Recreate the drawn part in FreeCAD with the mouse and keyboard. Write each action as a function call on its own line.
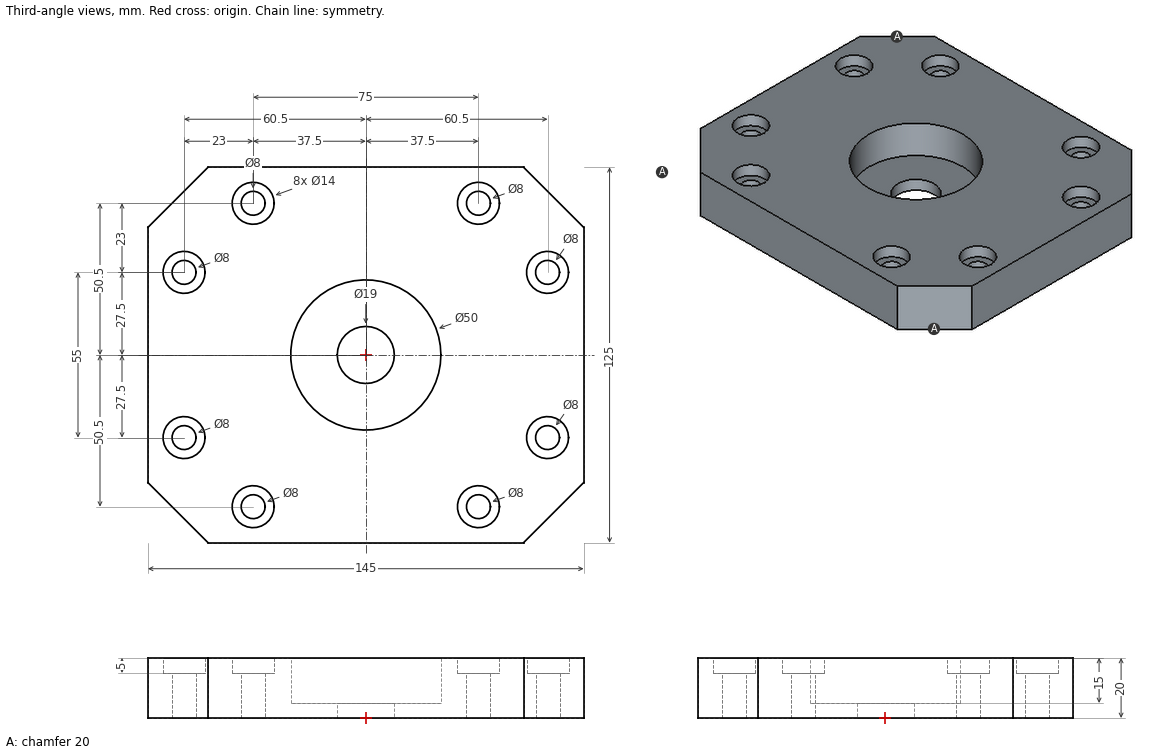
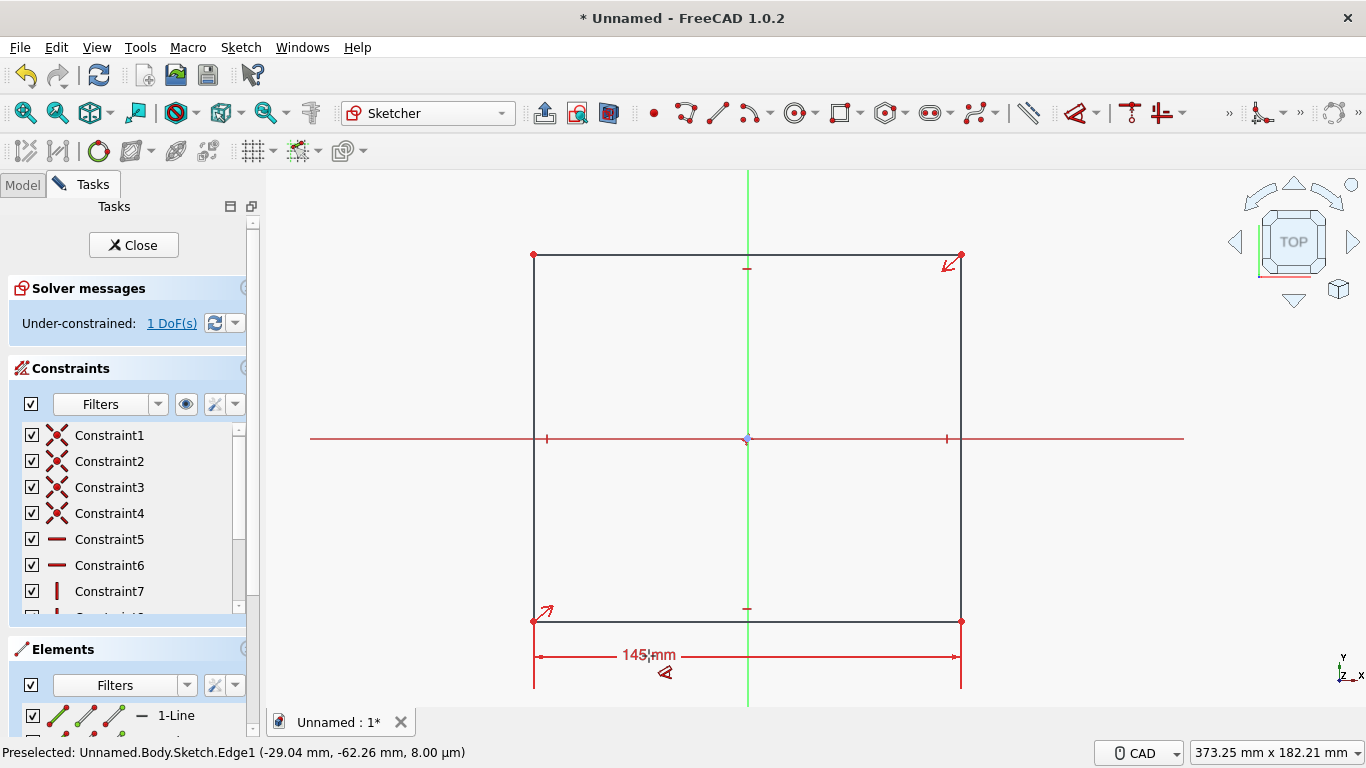
click(961, 512)
click(995, 354)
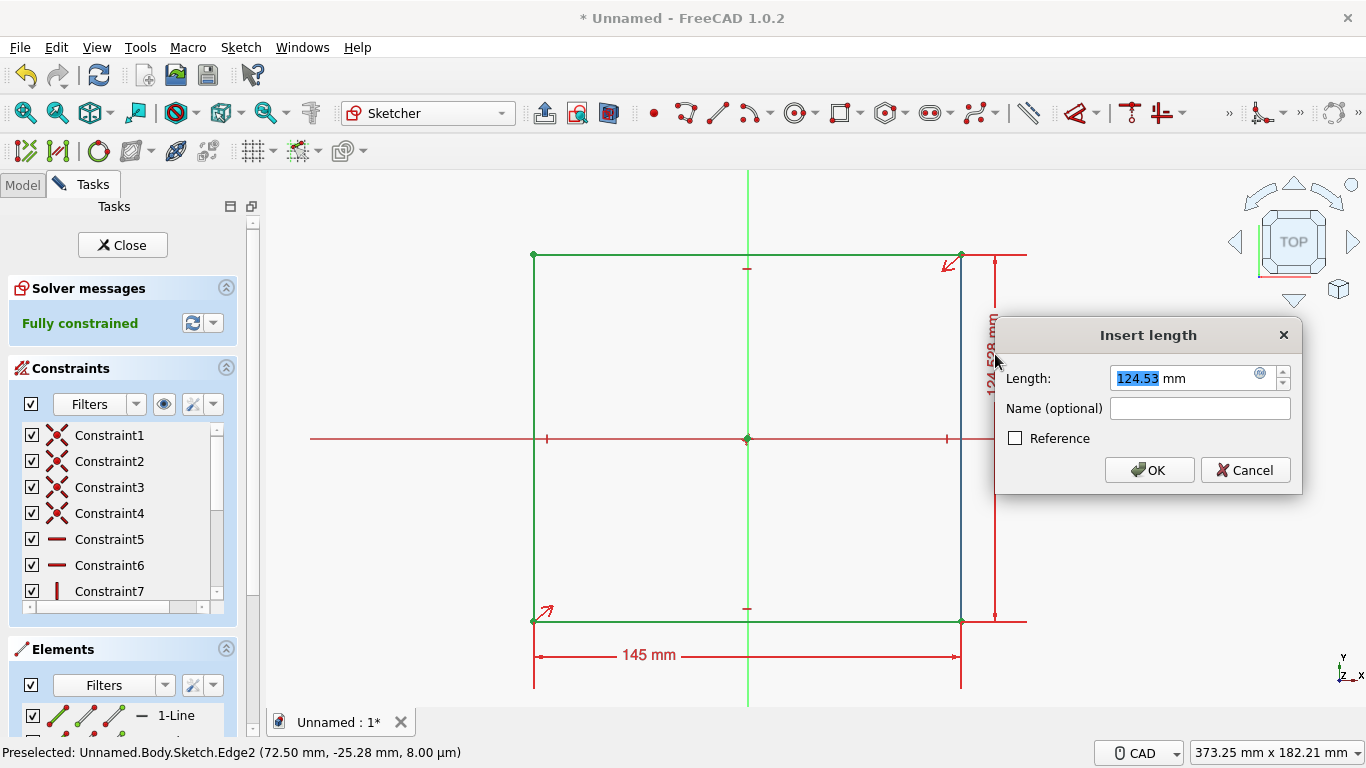
text(125)
key(Return)
key(Escape)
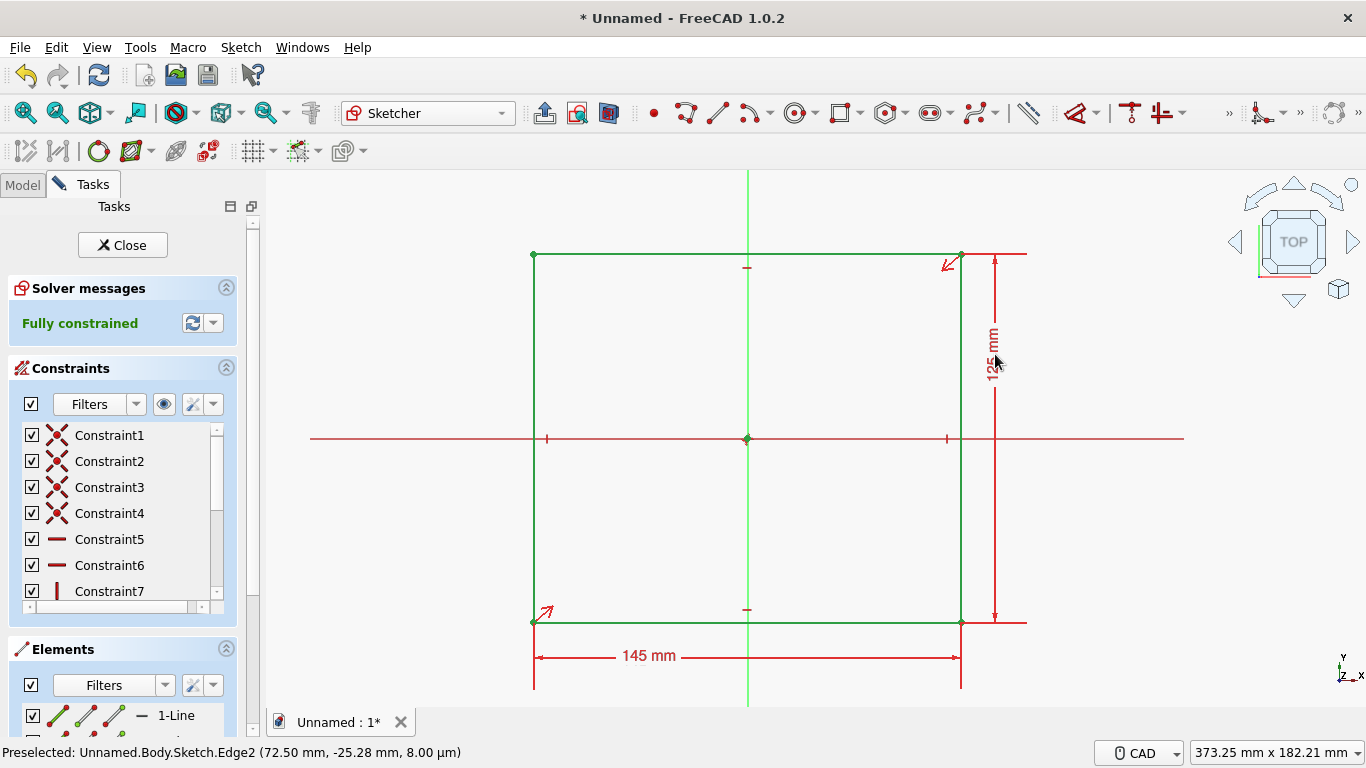
click(123, 245)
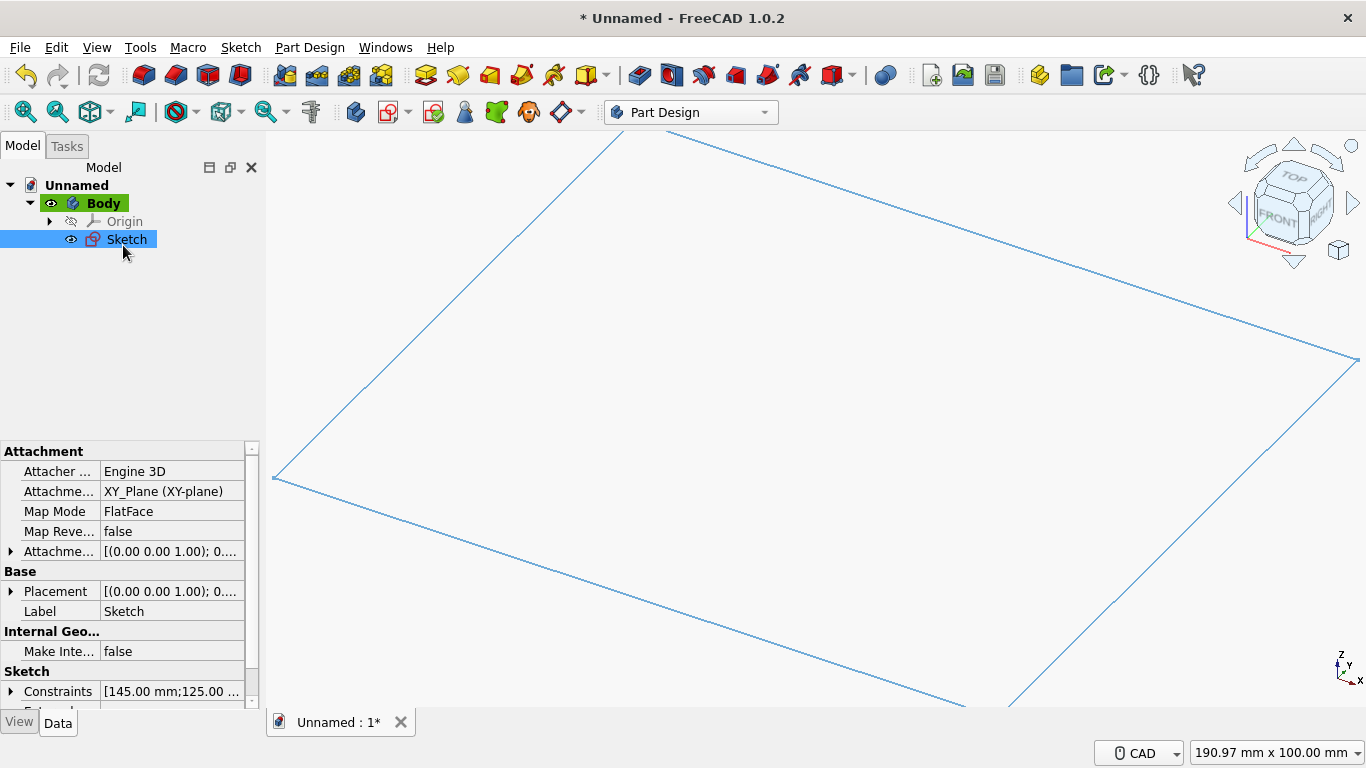
click(426, 76)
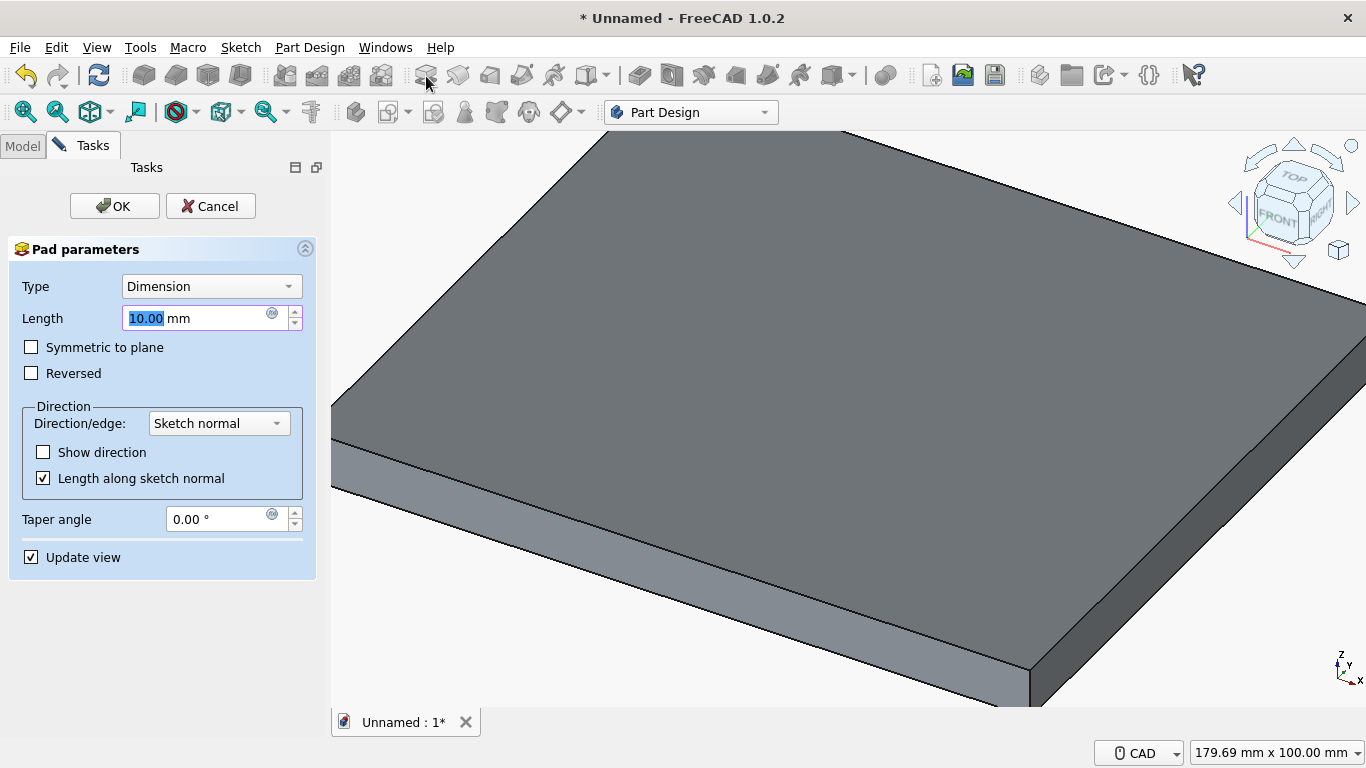
text(20)
key(Tab)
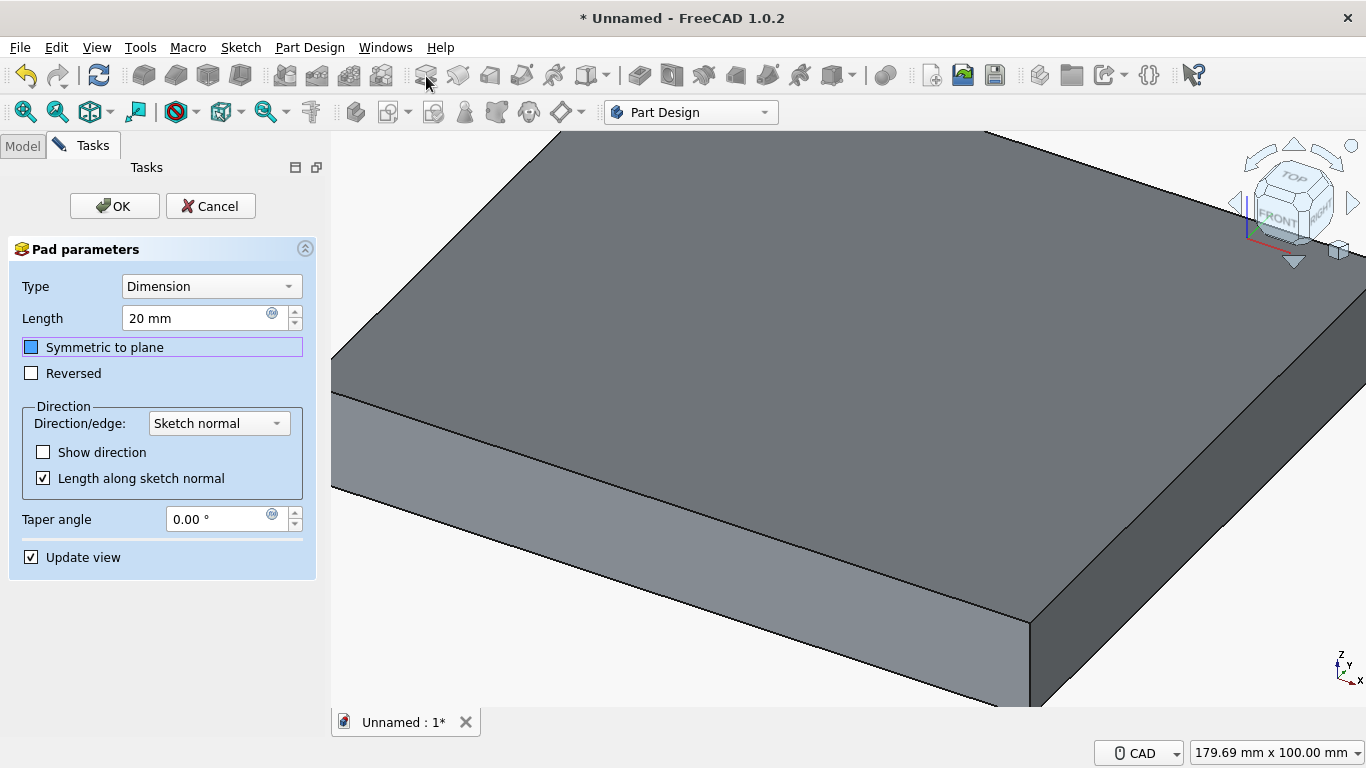
click(115, 206)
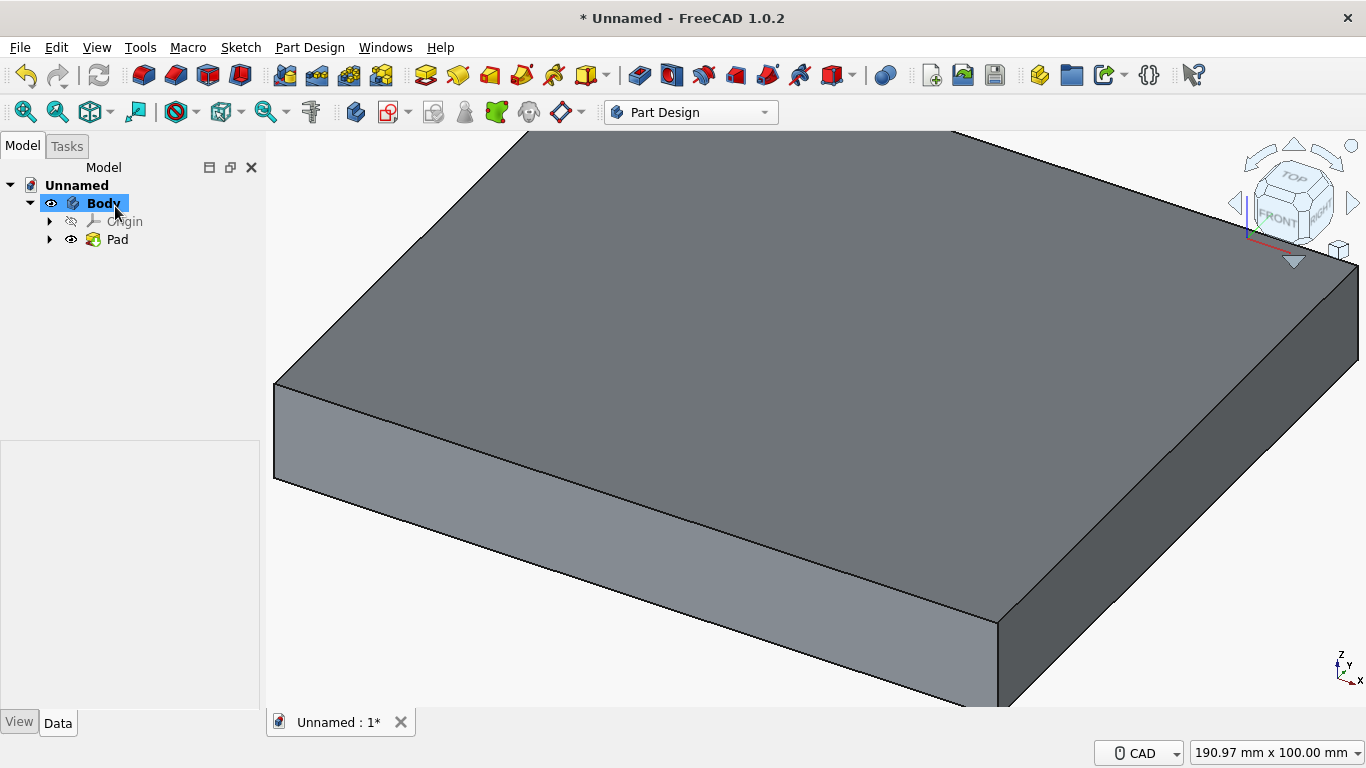
click(26, 112)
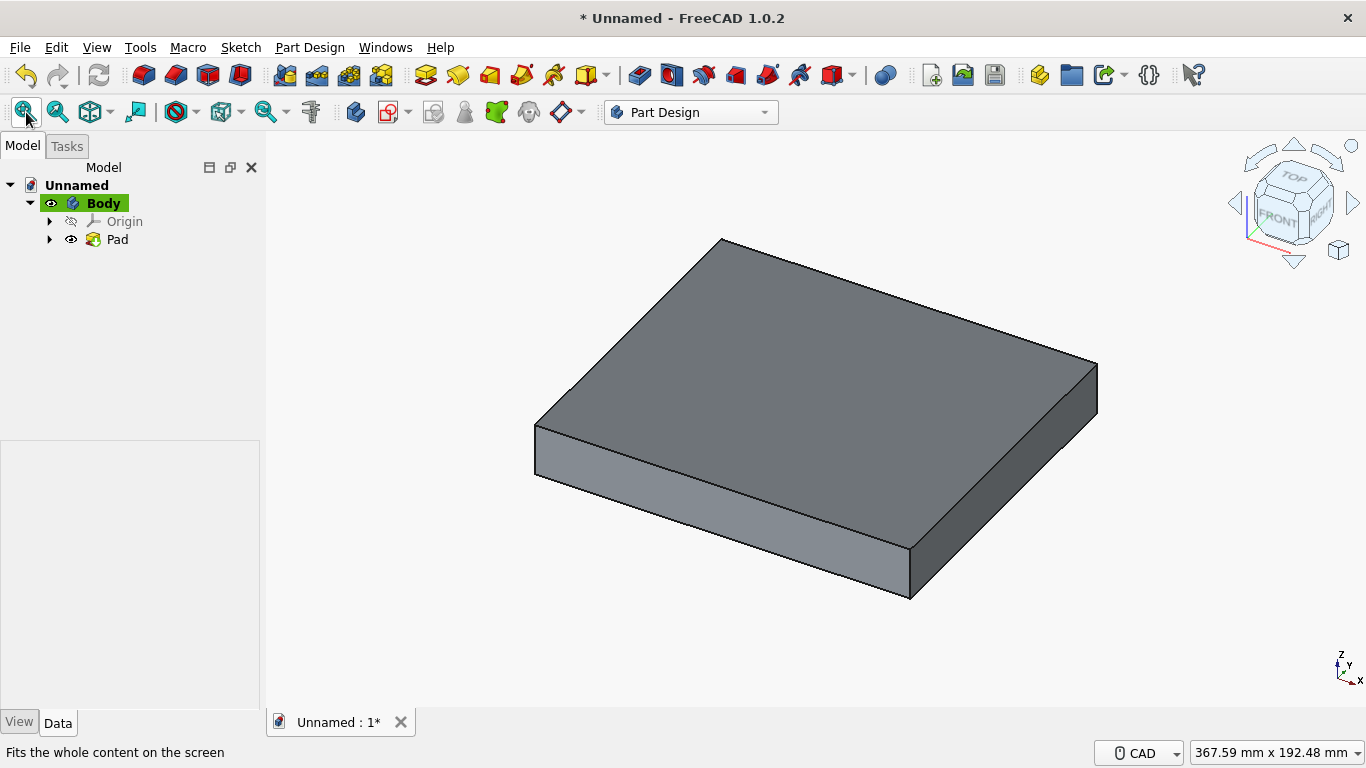
click(910, 573)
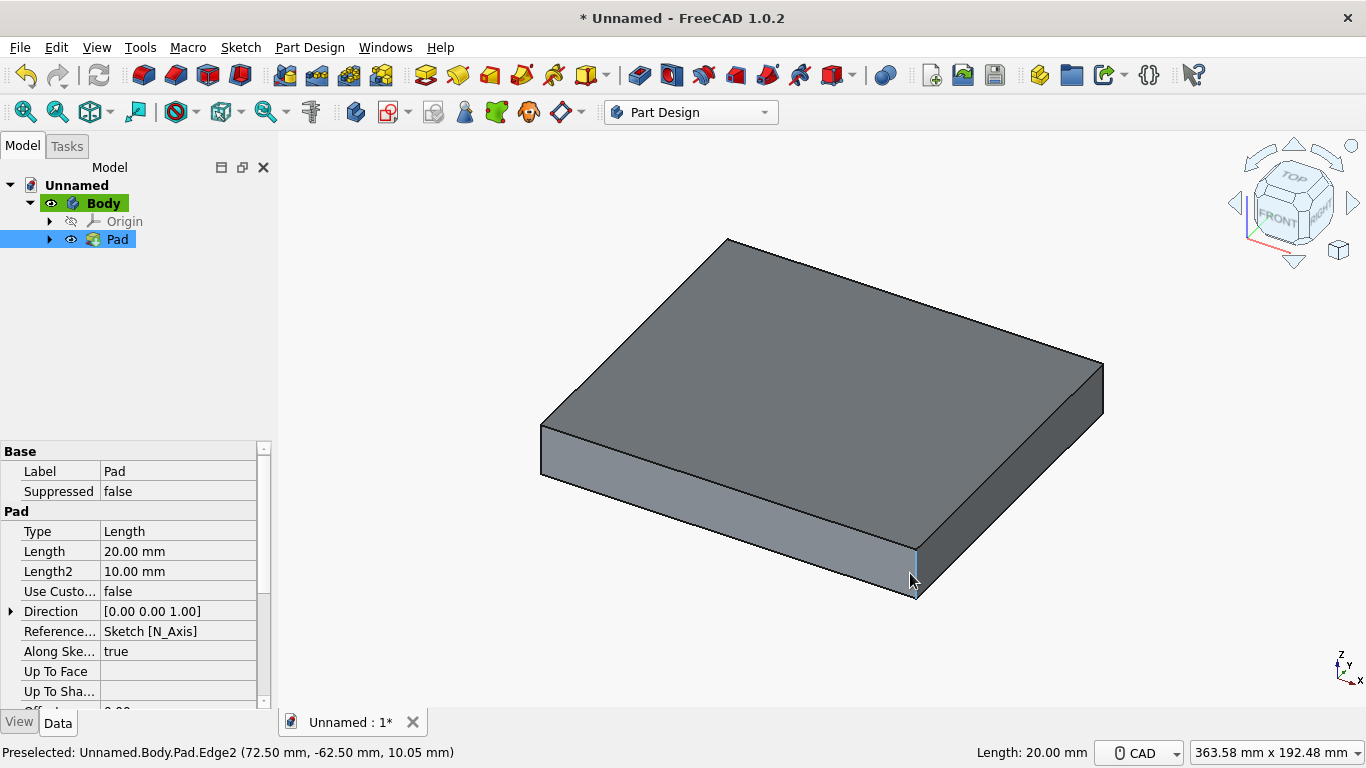
key(0)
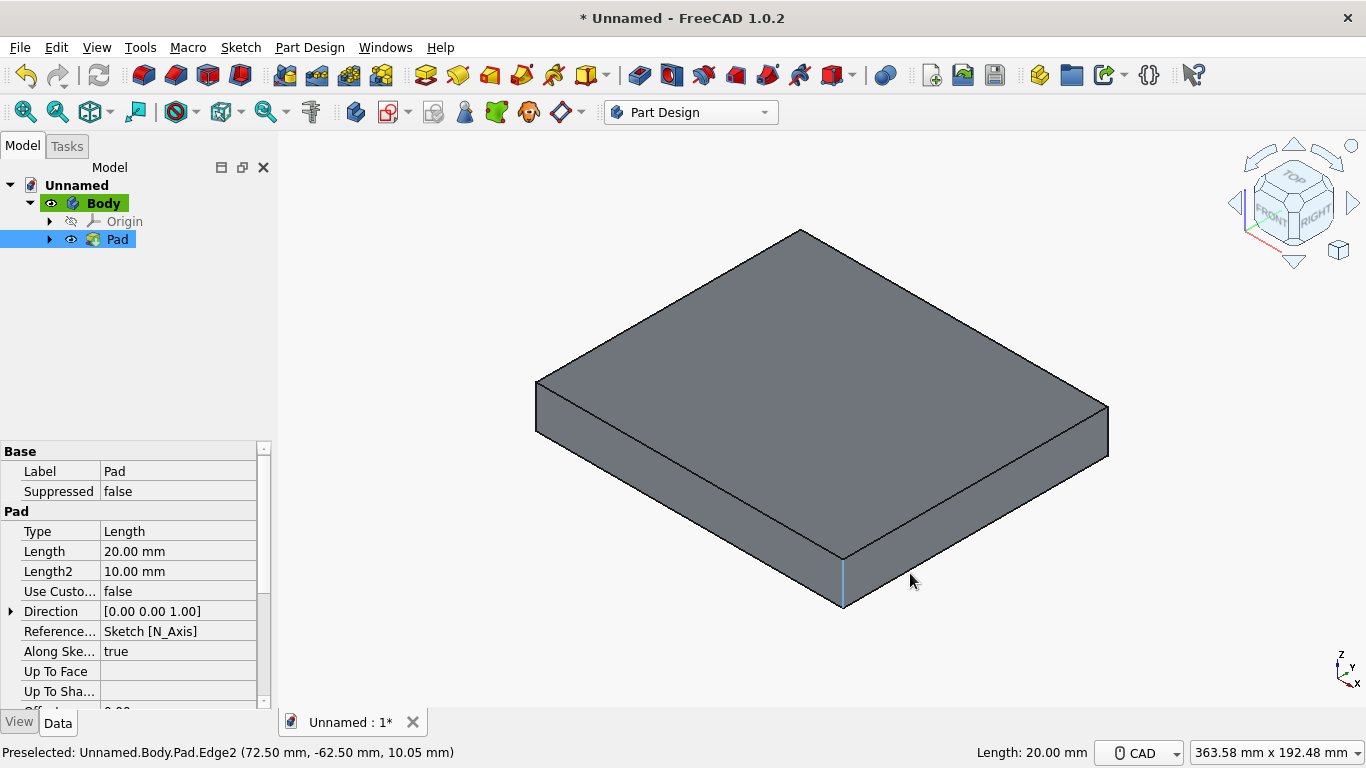
key(2)